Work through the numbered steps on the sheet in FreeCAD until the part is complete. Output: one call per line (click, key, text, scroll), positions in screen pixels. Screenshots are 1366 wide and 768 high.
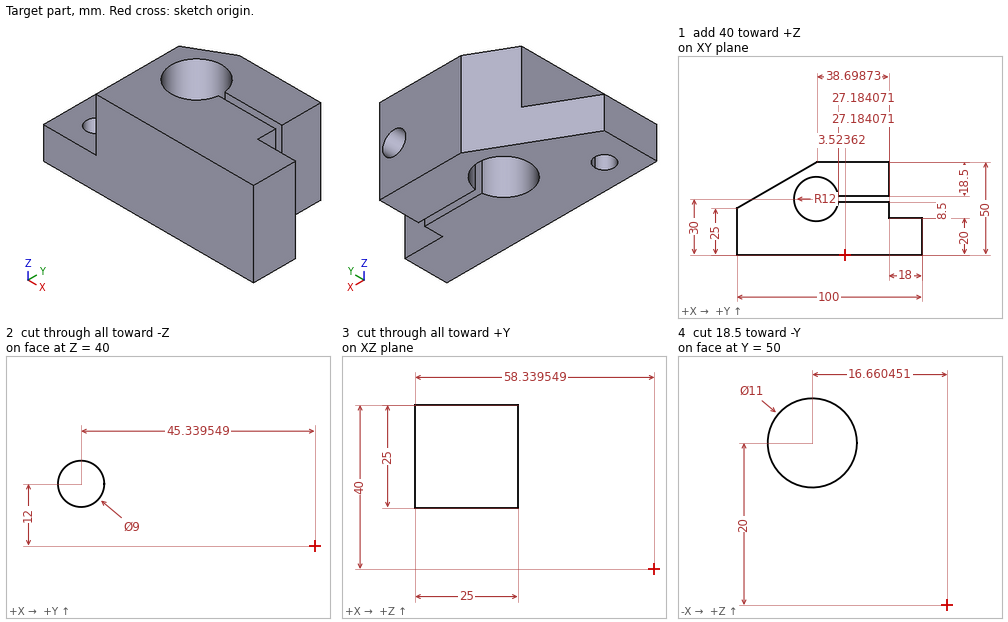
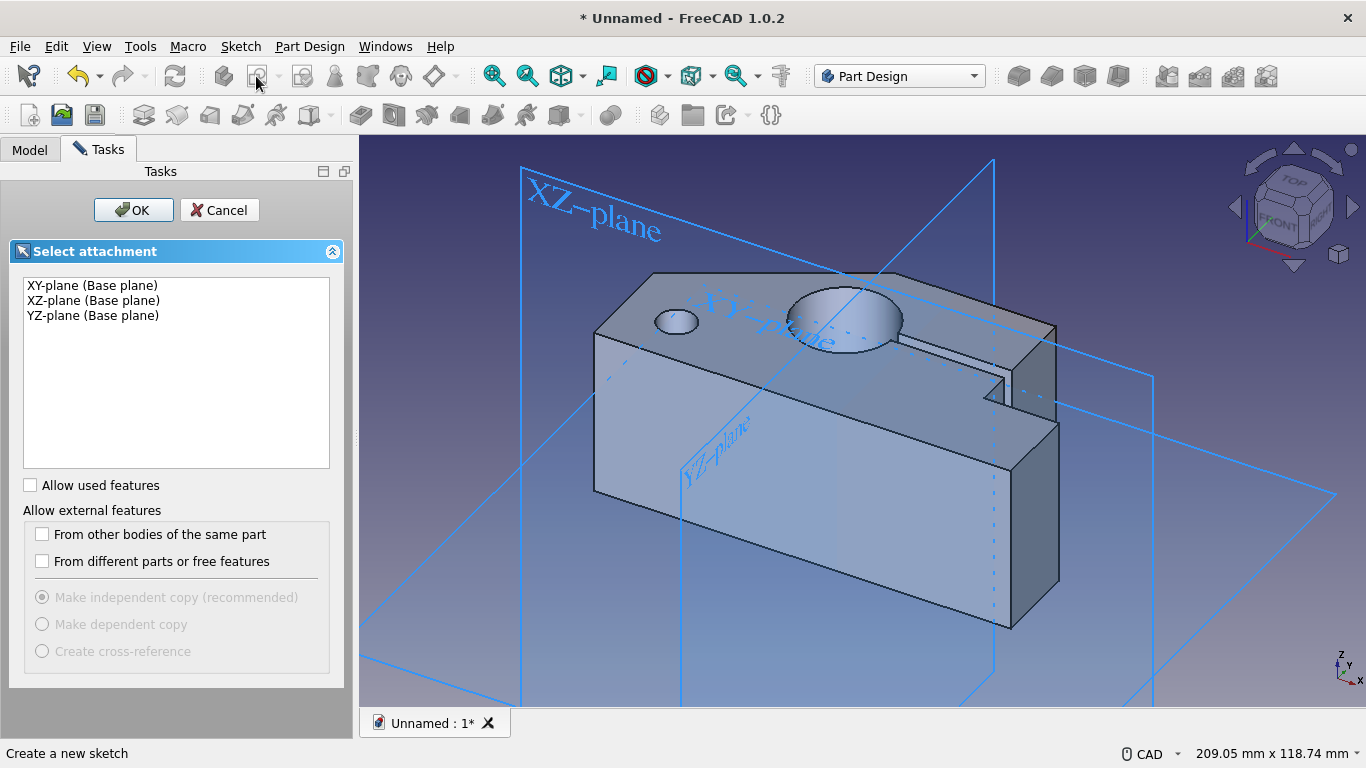
click(84, 300)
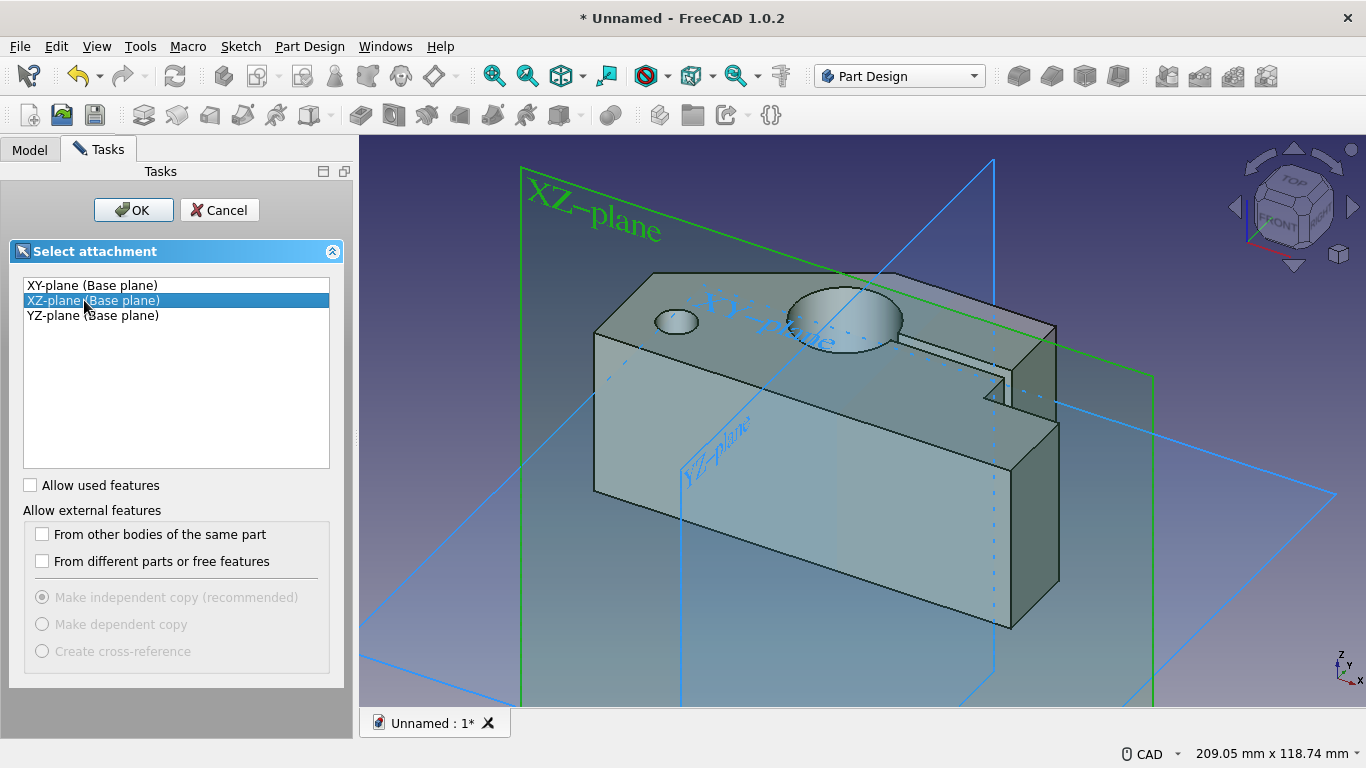
click(134, 210)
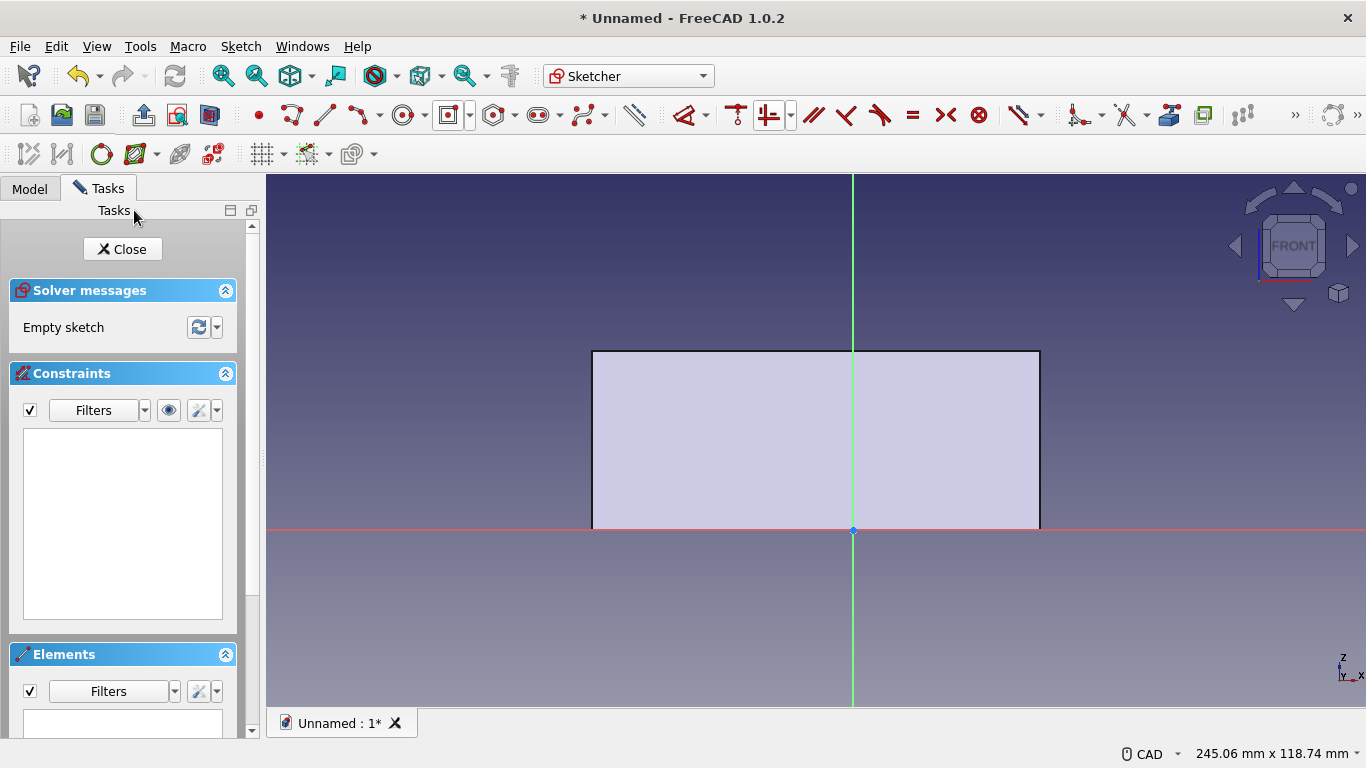
scroll(692, 441, up, 3)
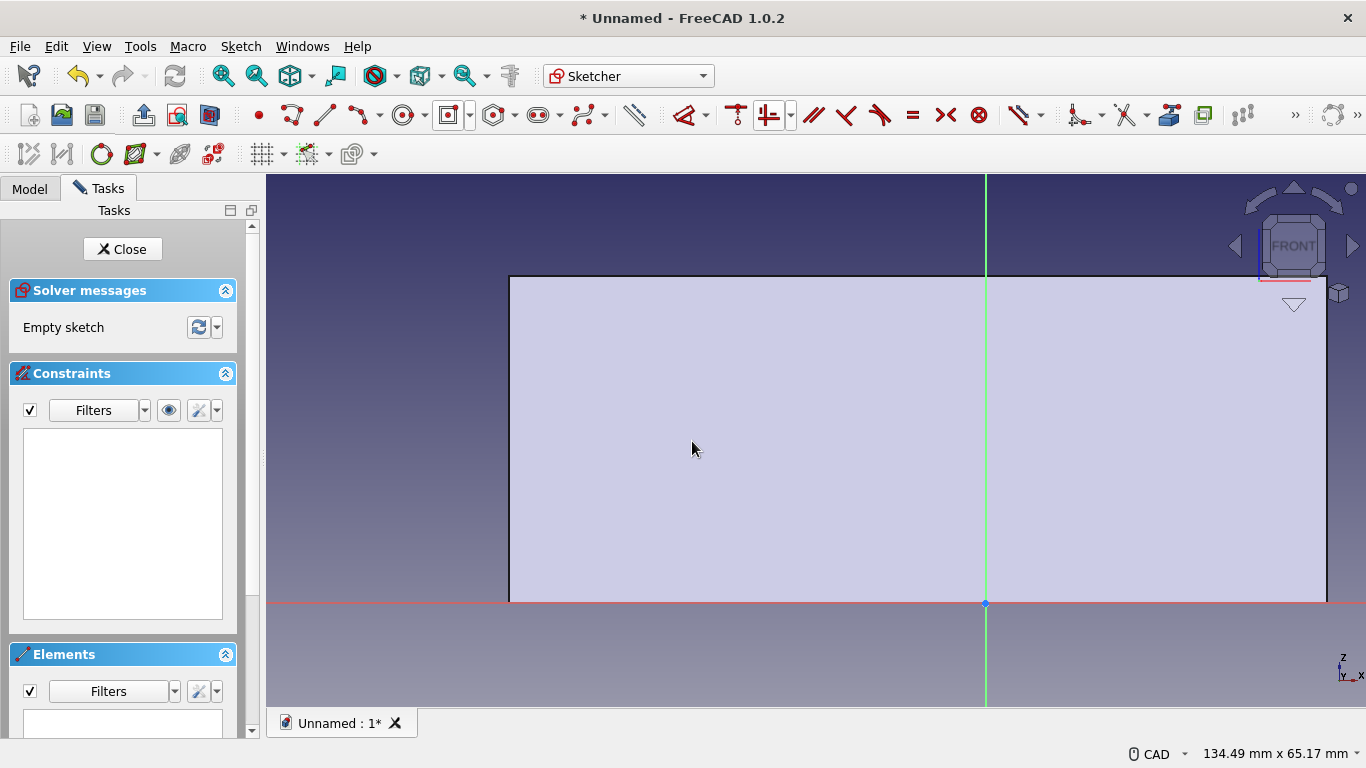
key(g)
key(r)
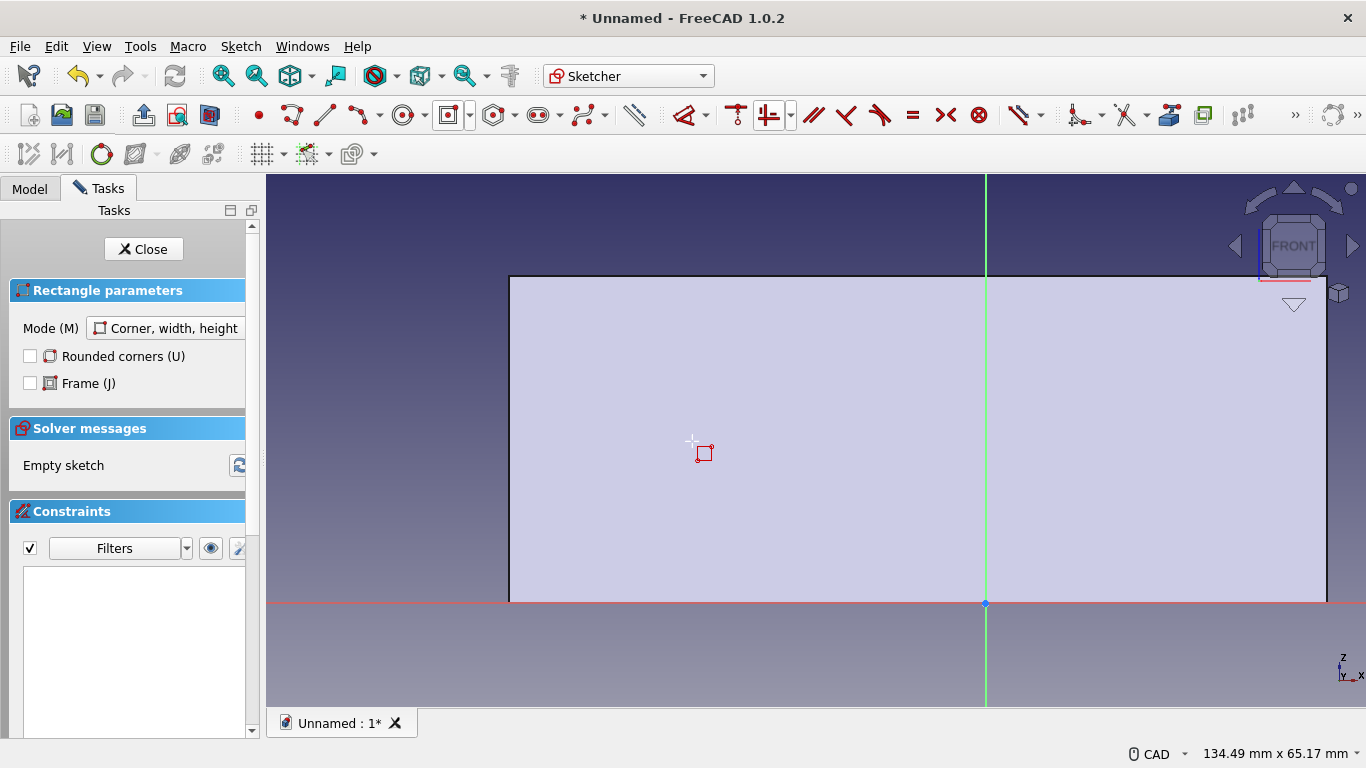
click(509, 276)
move(713, 481)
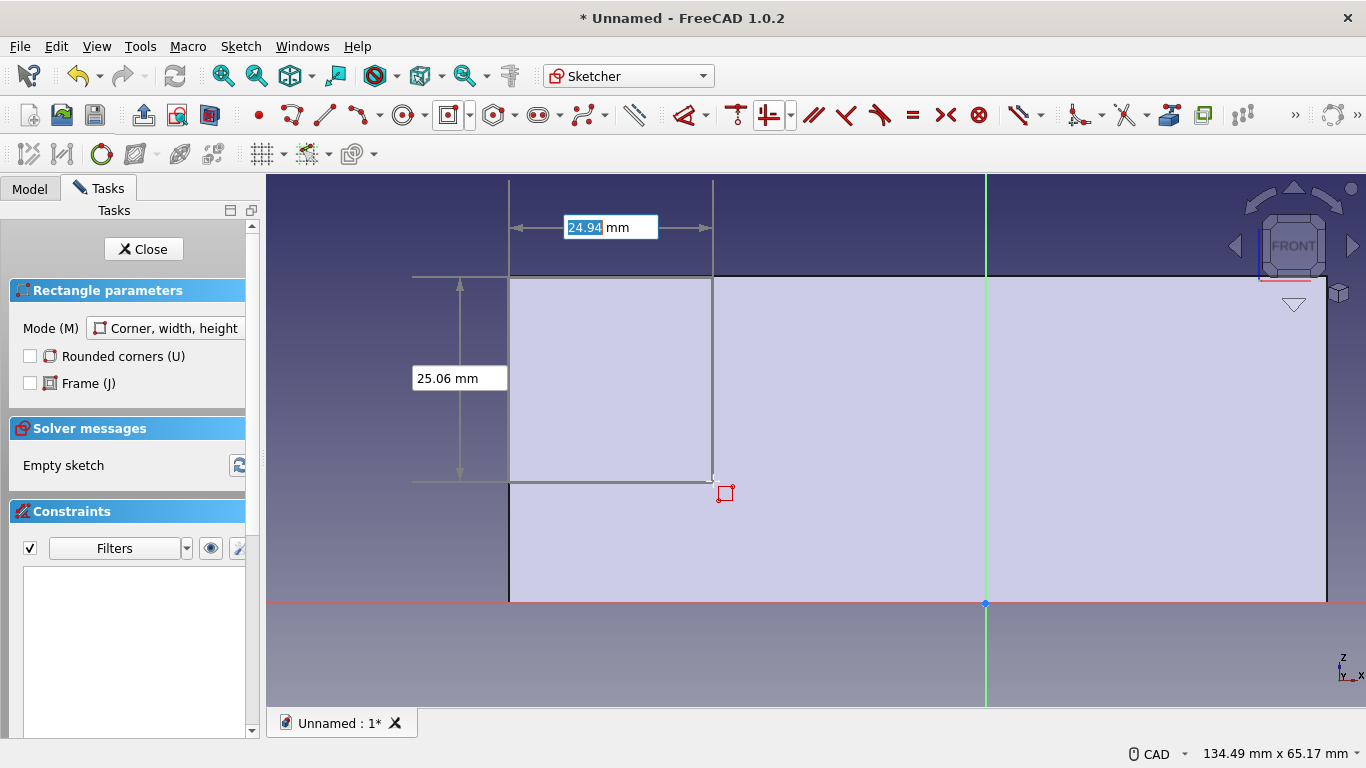
text(25)
key(Tab)
text(25)
key(Return)
key(Escape)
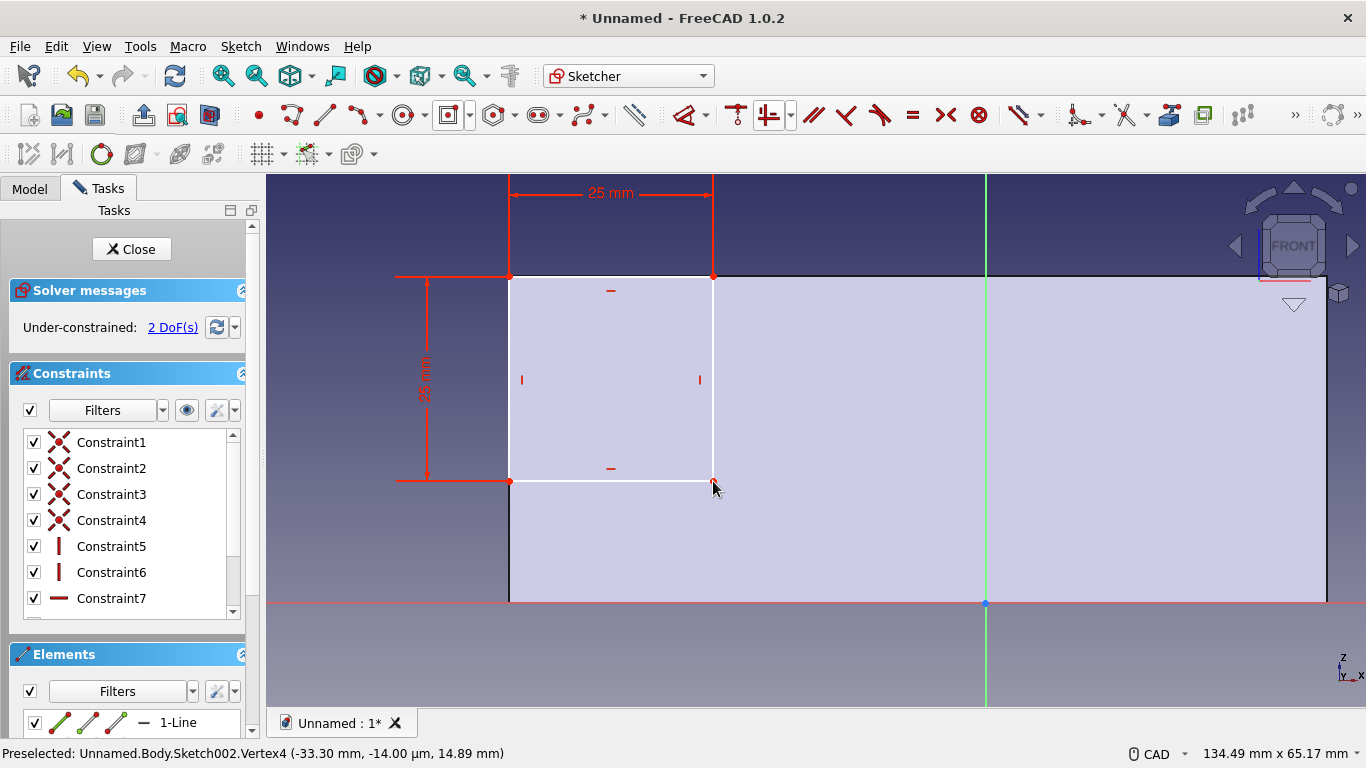
click(684, 116)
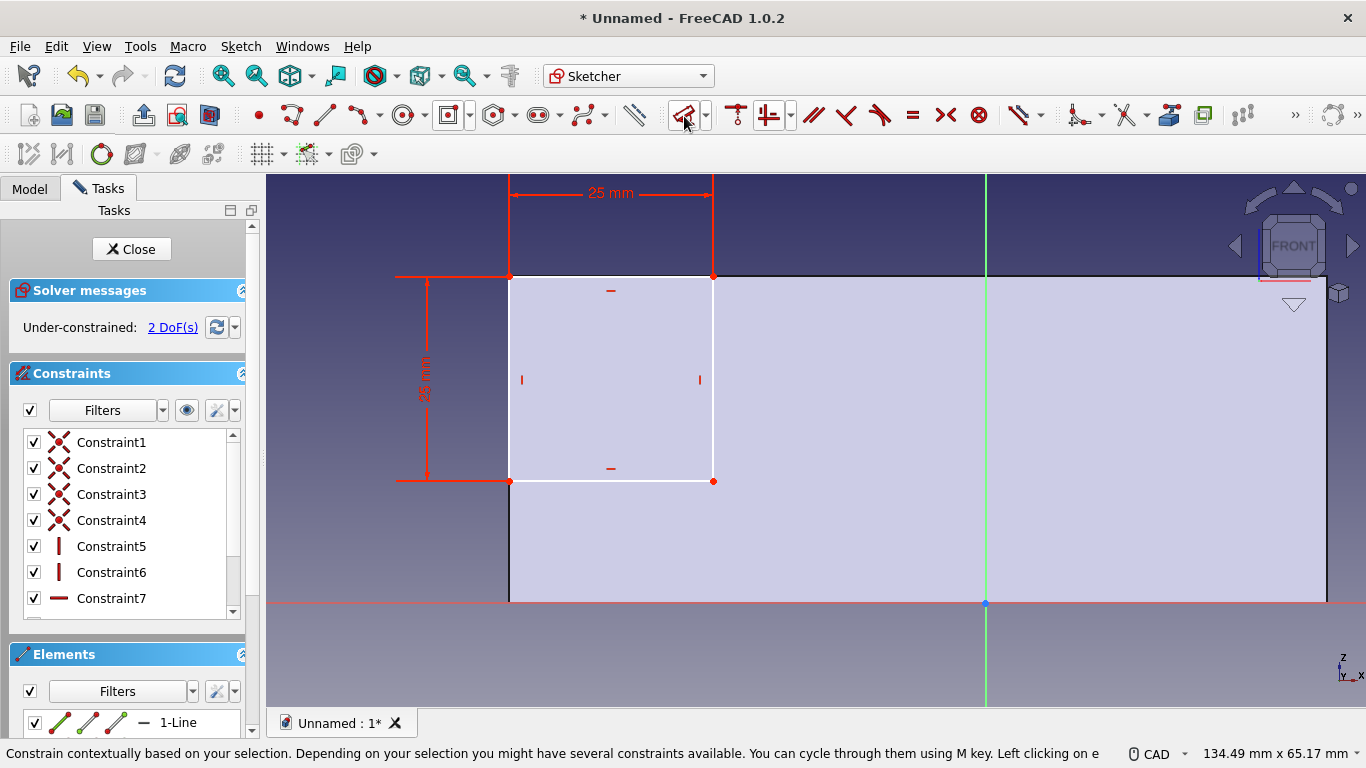
click(509, 277)
click(1020, 440)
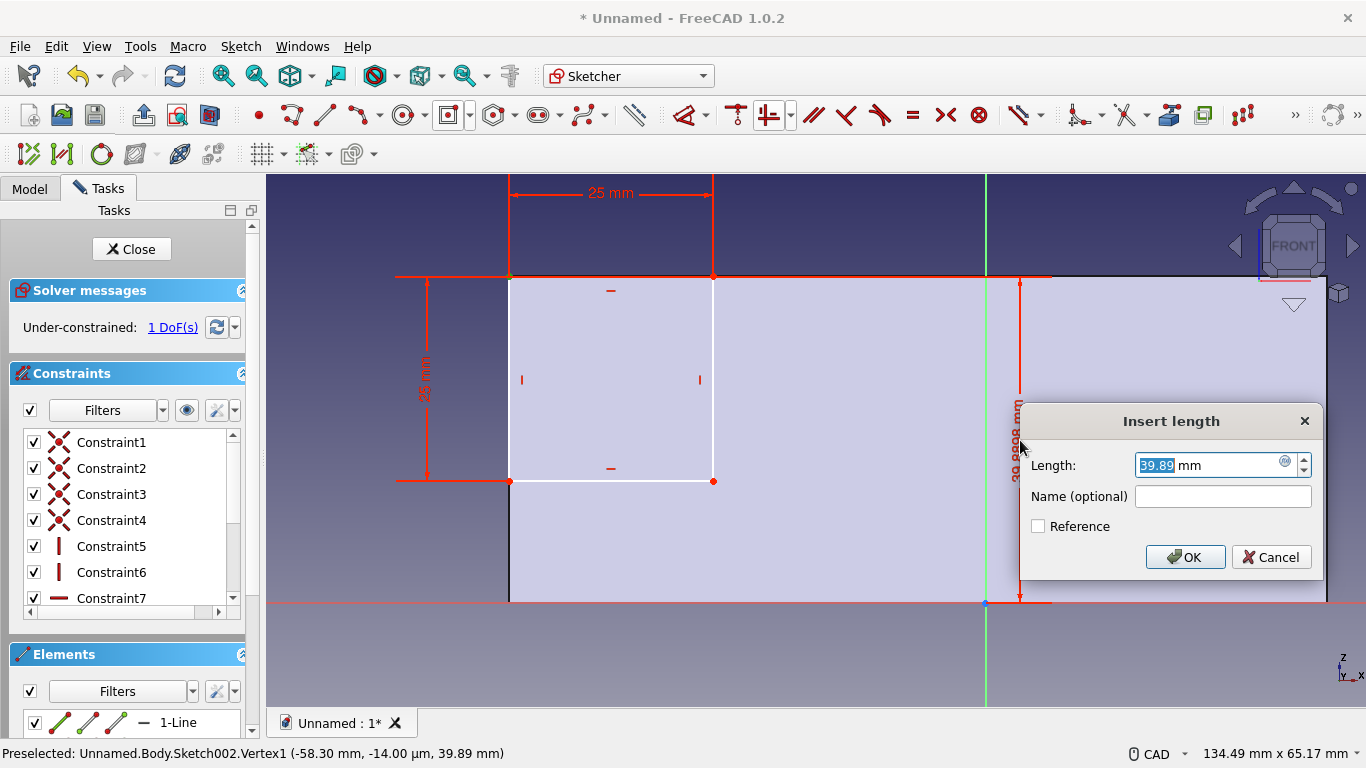
text(40)
key(Return)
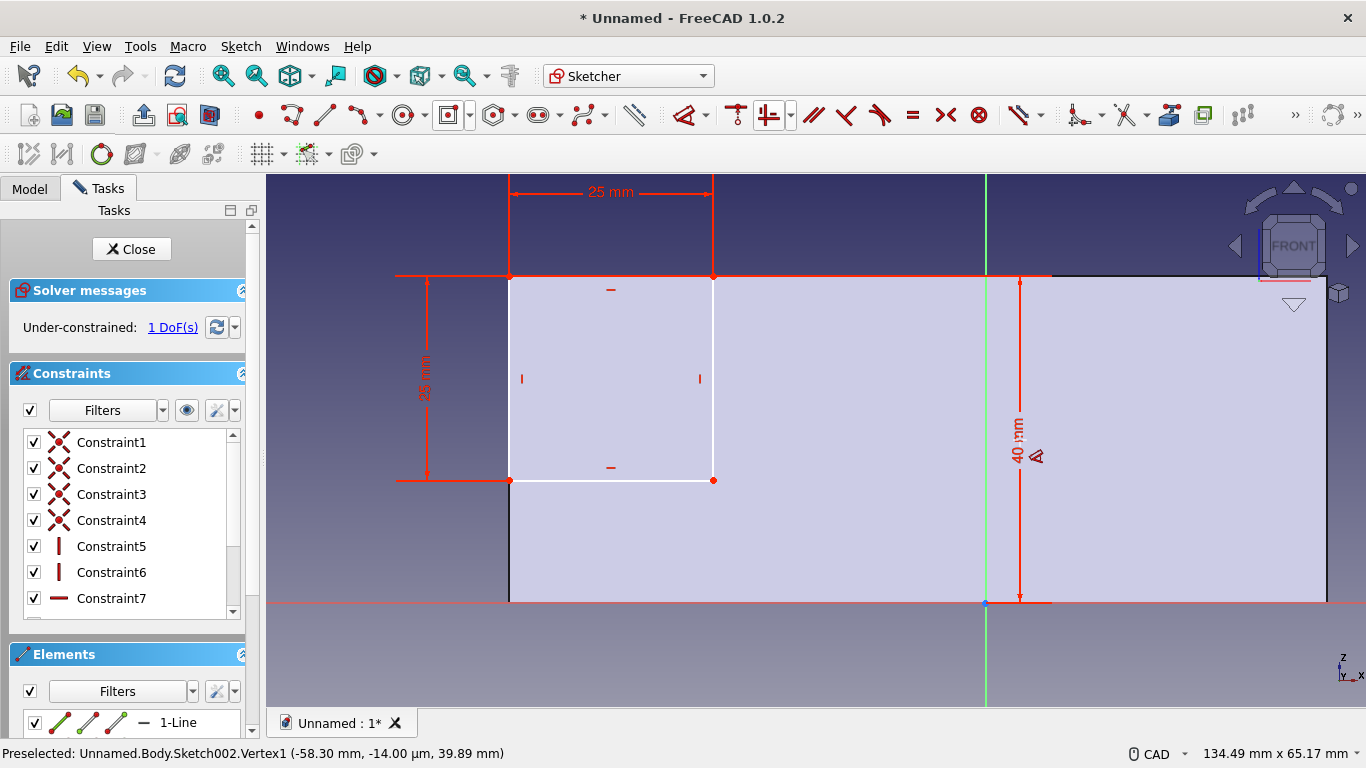
click(509, 276)
click(747, 637)